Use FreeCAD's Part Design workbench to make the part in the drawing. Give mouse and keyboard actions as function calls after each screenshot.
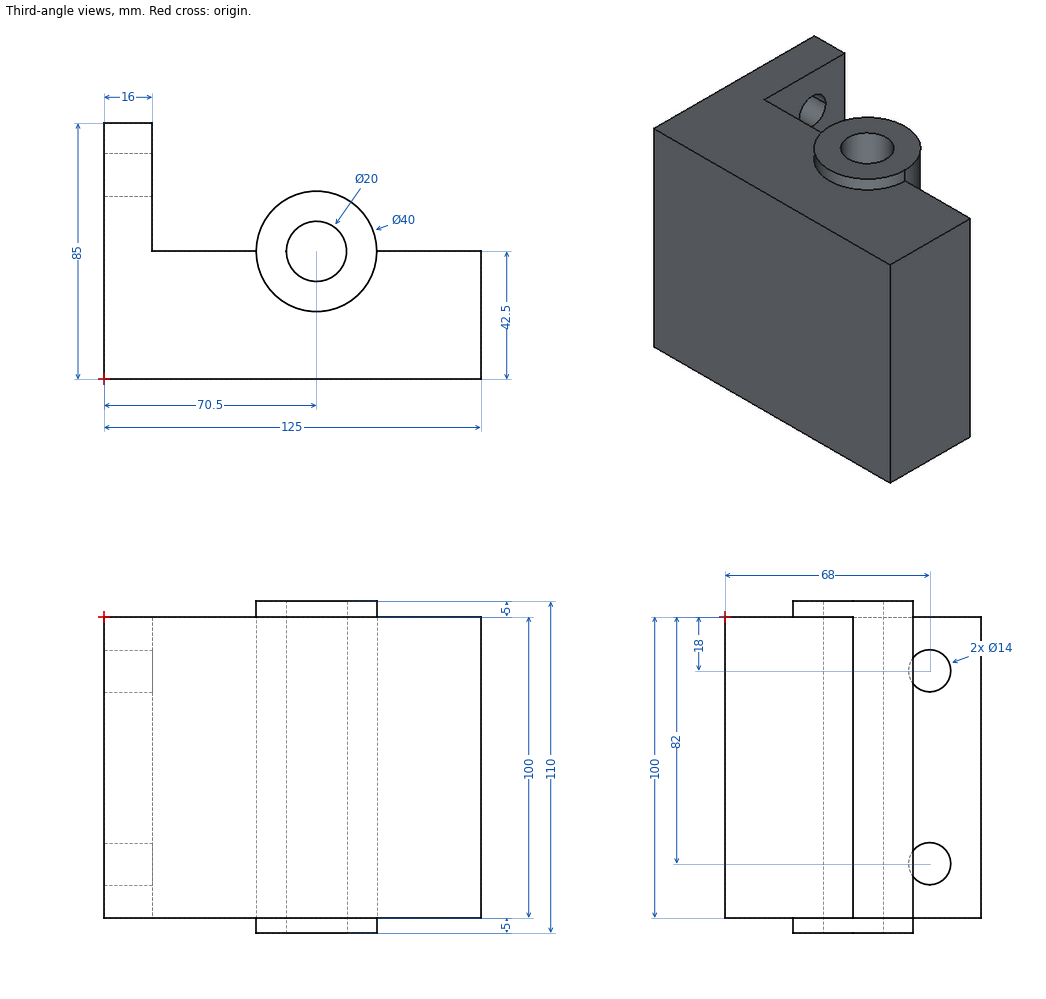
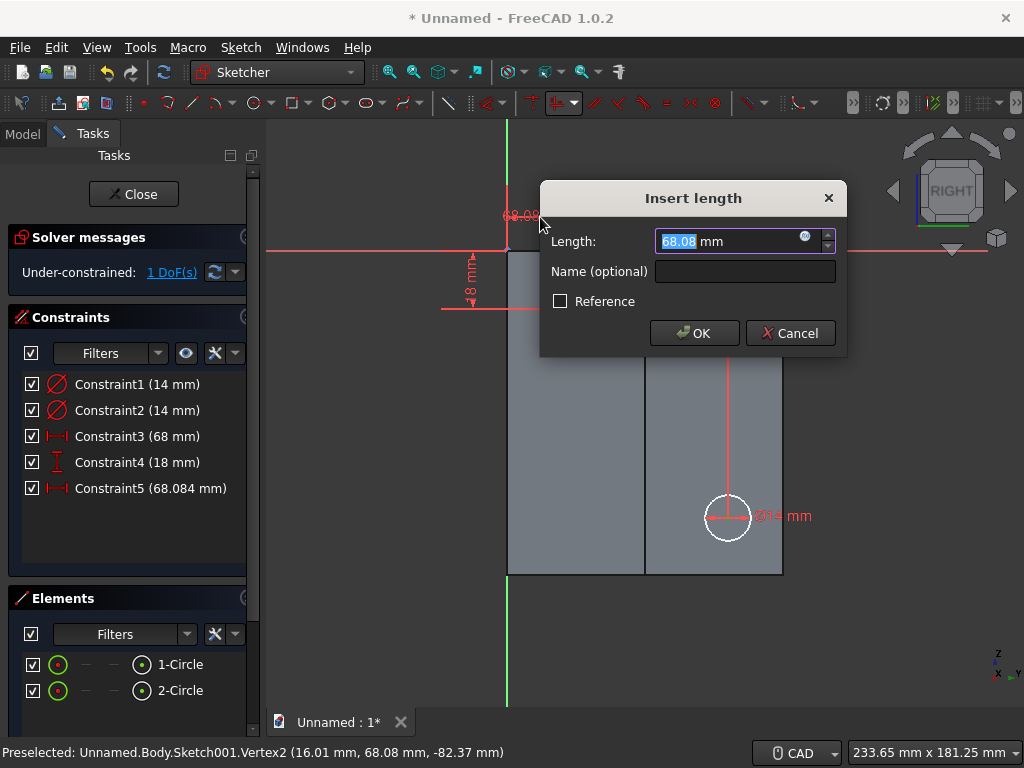
text(68)
key(Return)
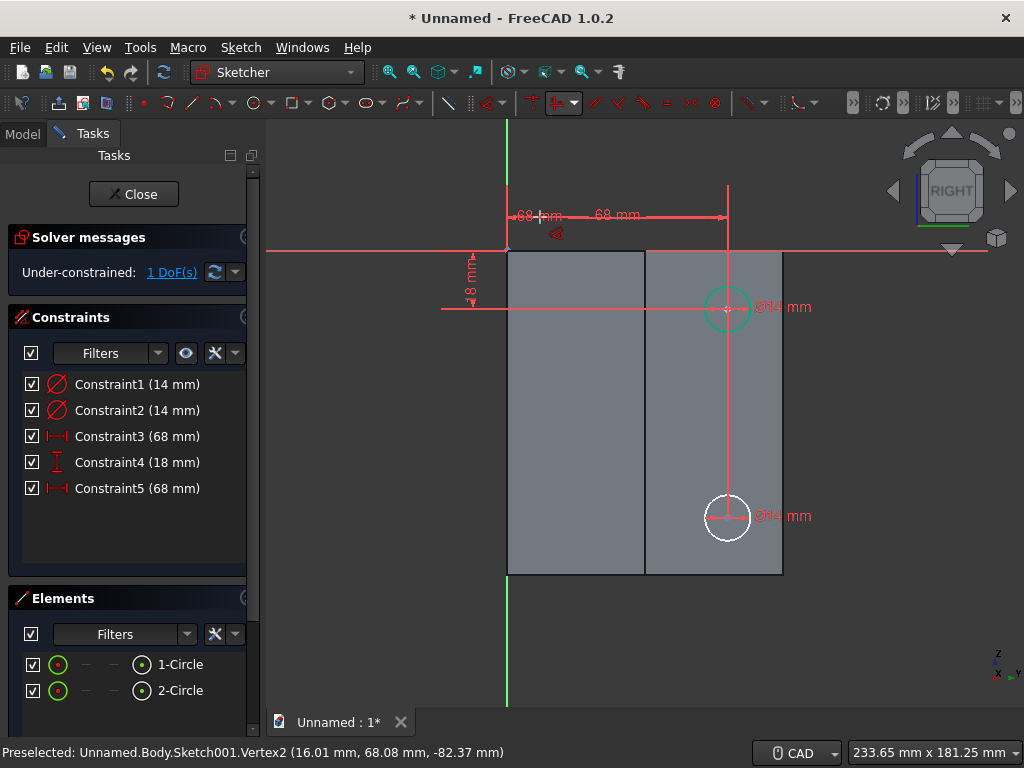
click(728, 518)
click(473, 384)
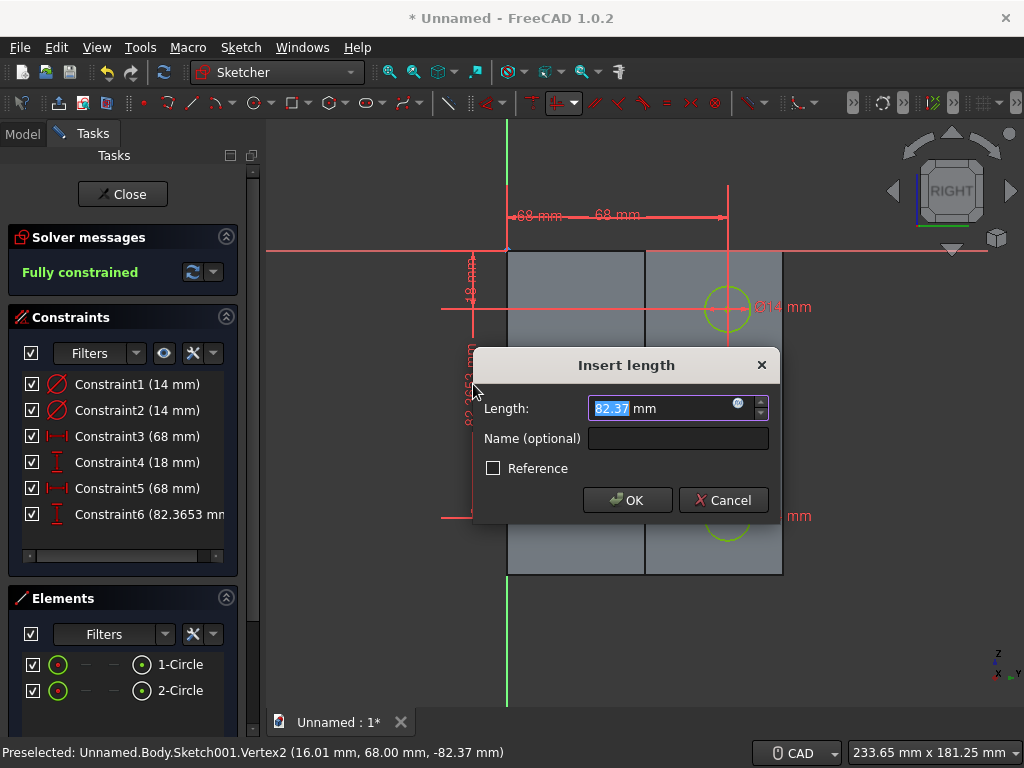
text(82)
key(Return)
key(Escape)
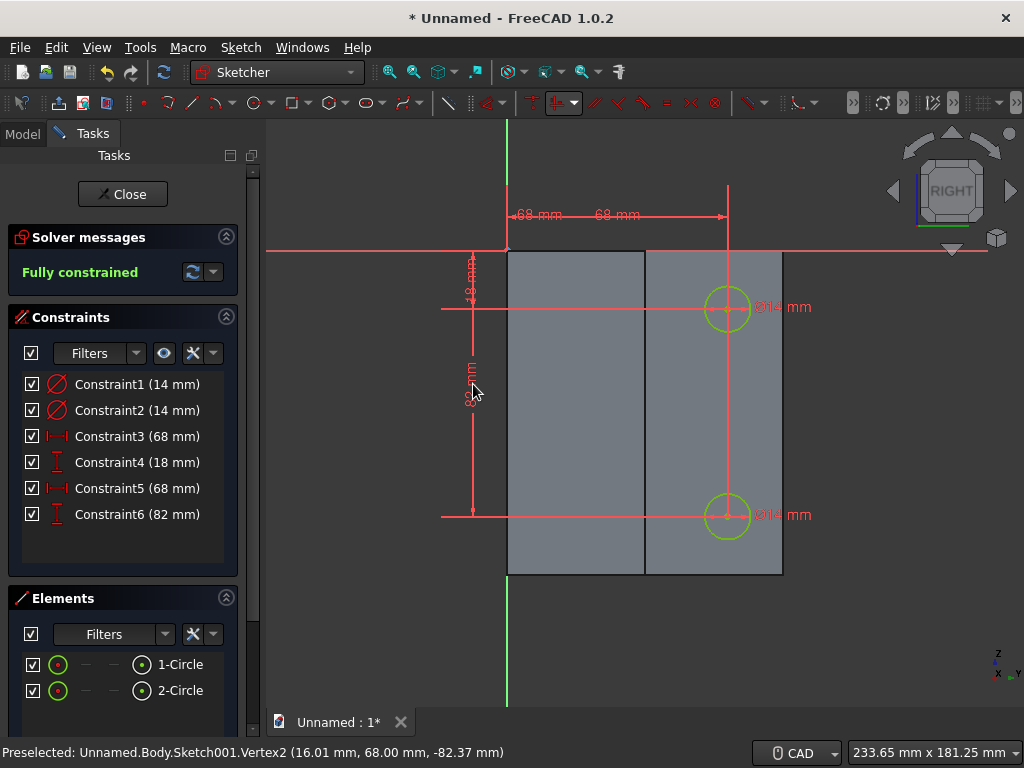
click(123, 194)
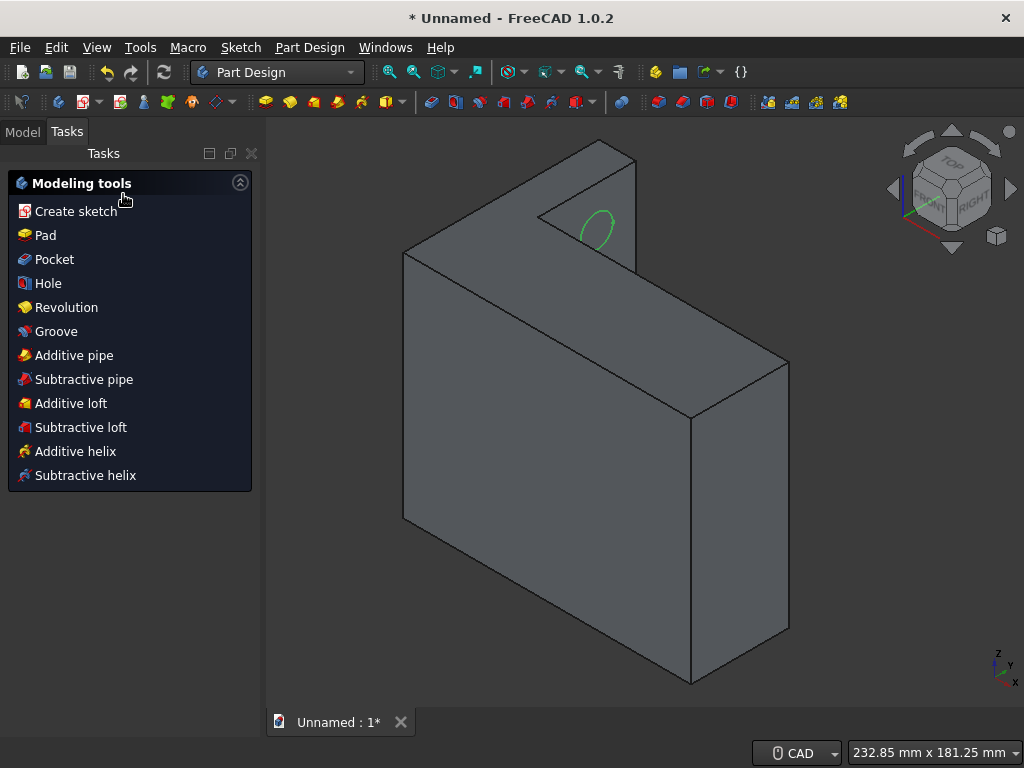
click(432, 102)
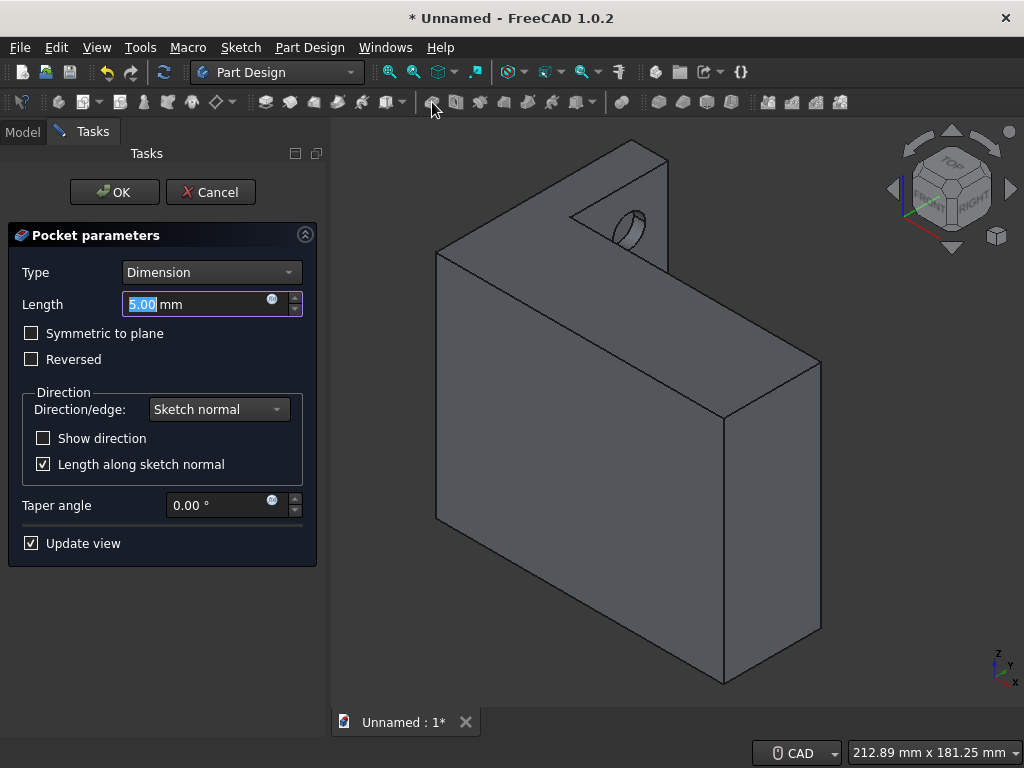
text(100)
key(Tab)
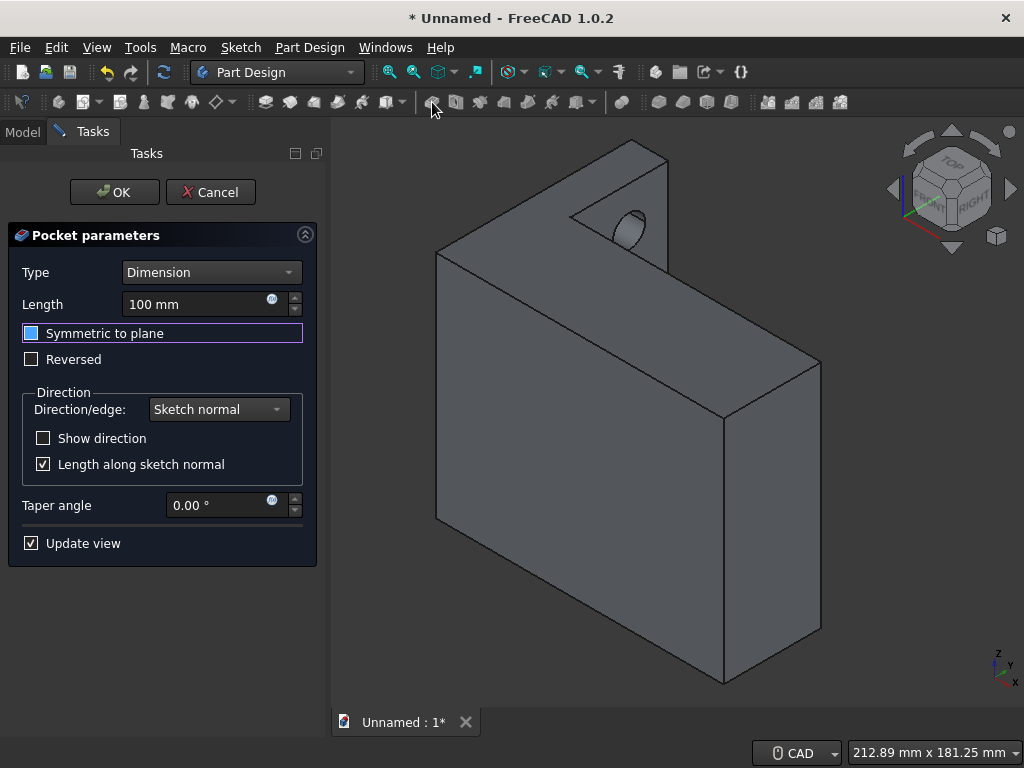
click(115, 192)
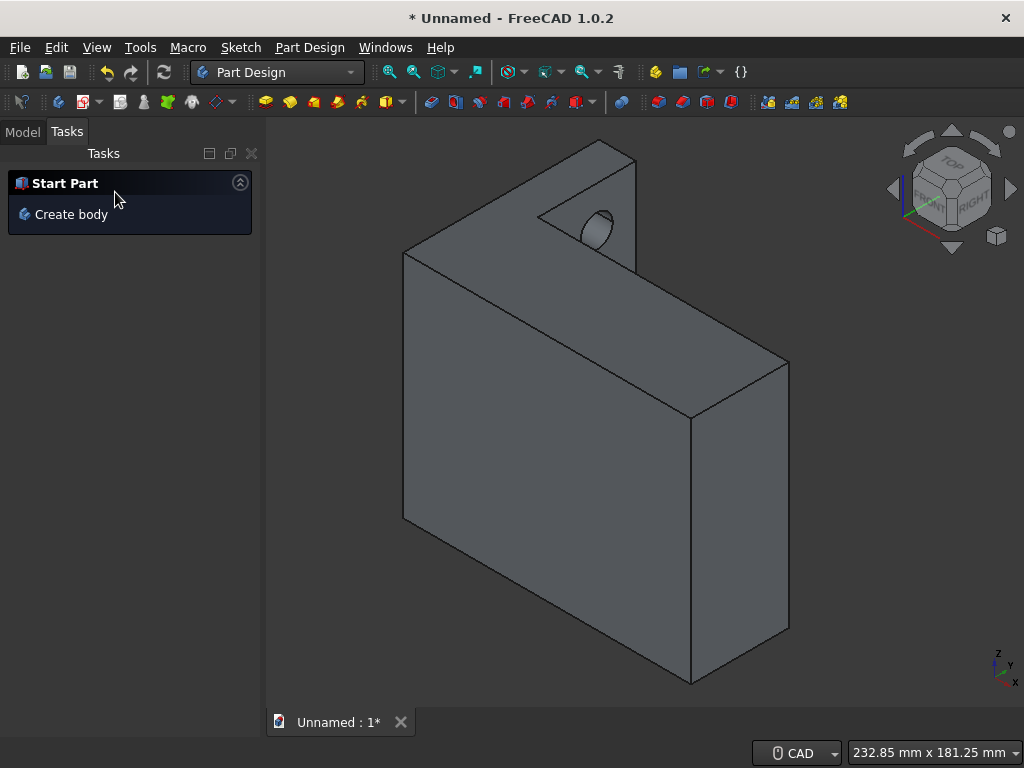
click(84, 102)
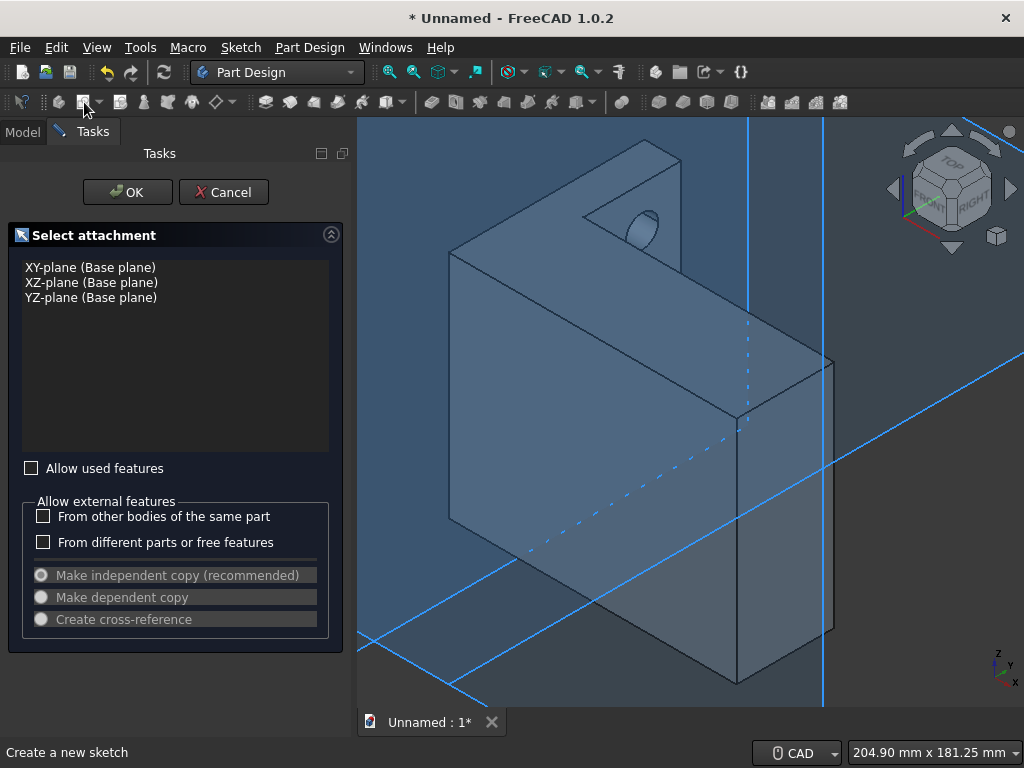
click(82, 268)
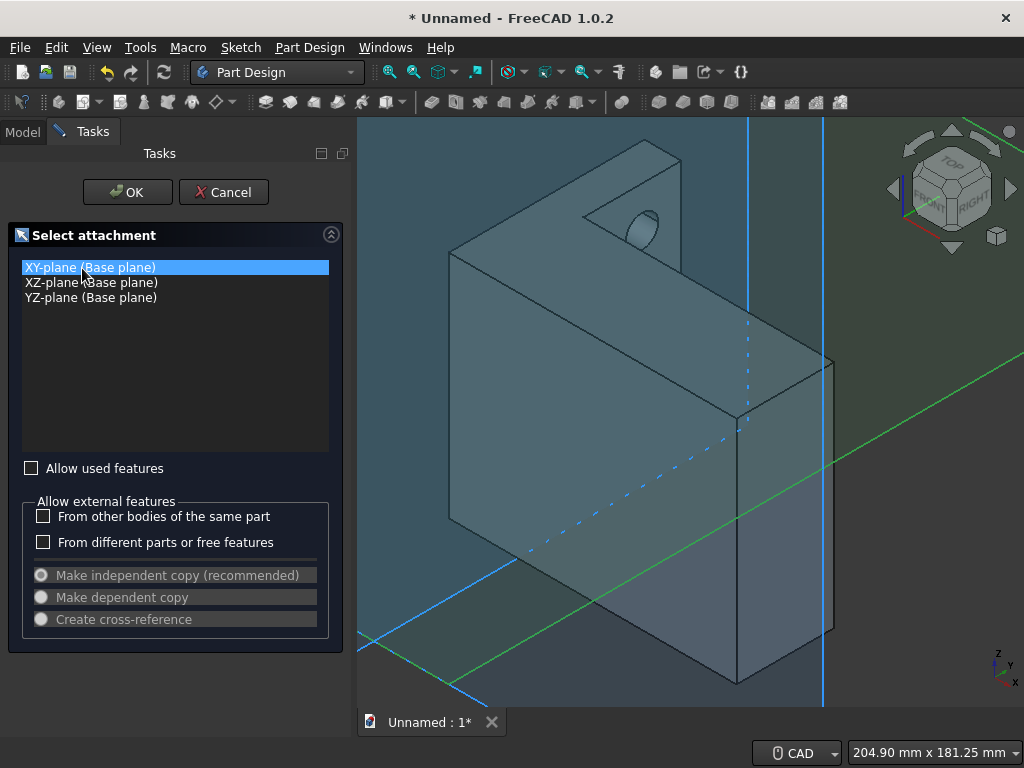
click(128, 192)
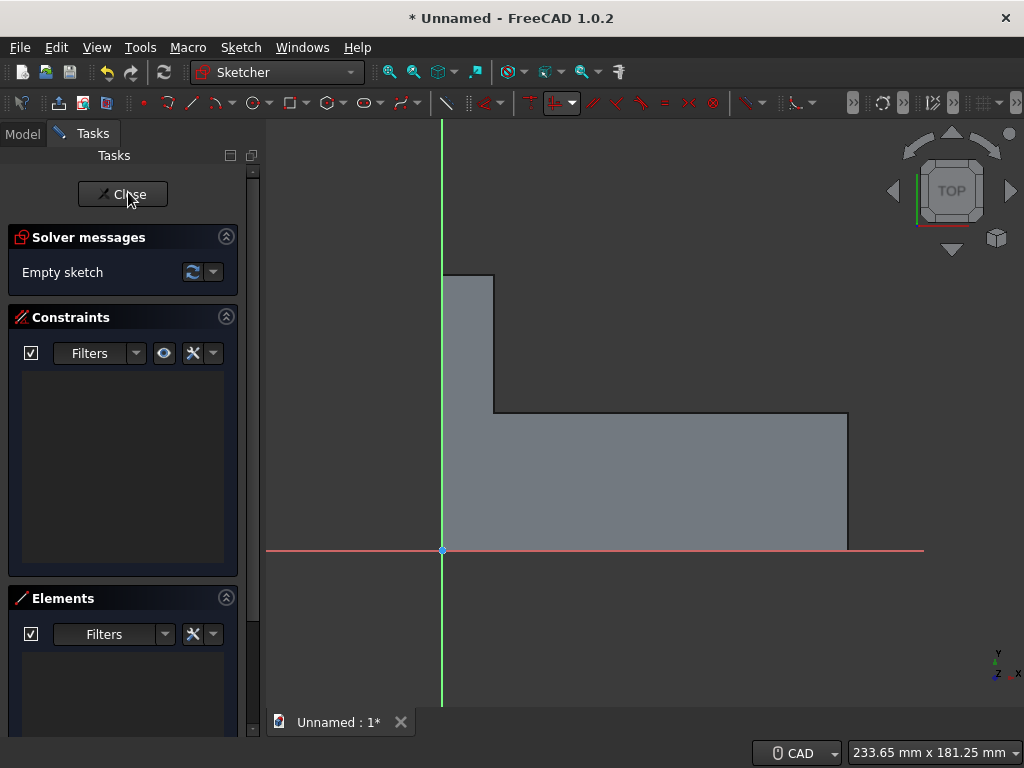
scroll(615, 524, up, 2)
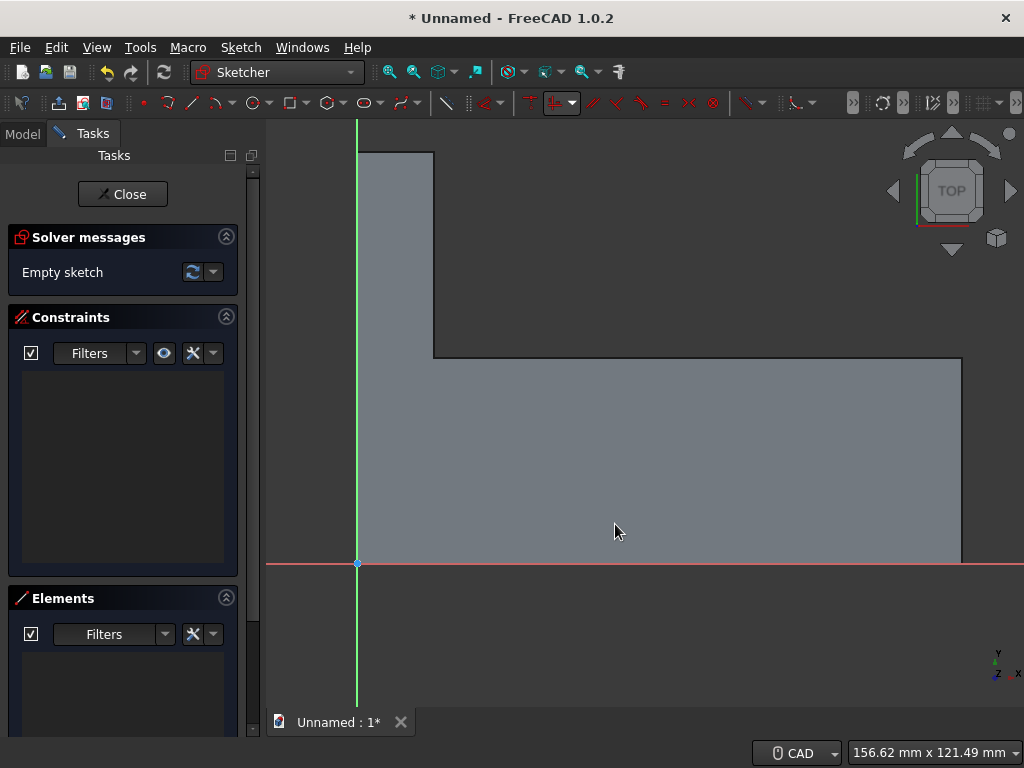
key(g)
key(c)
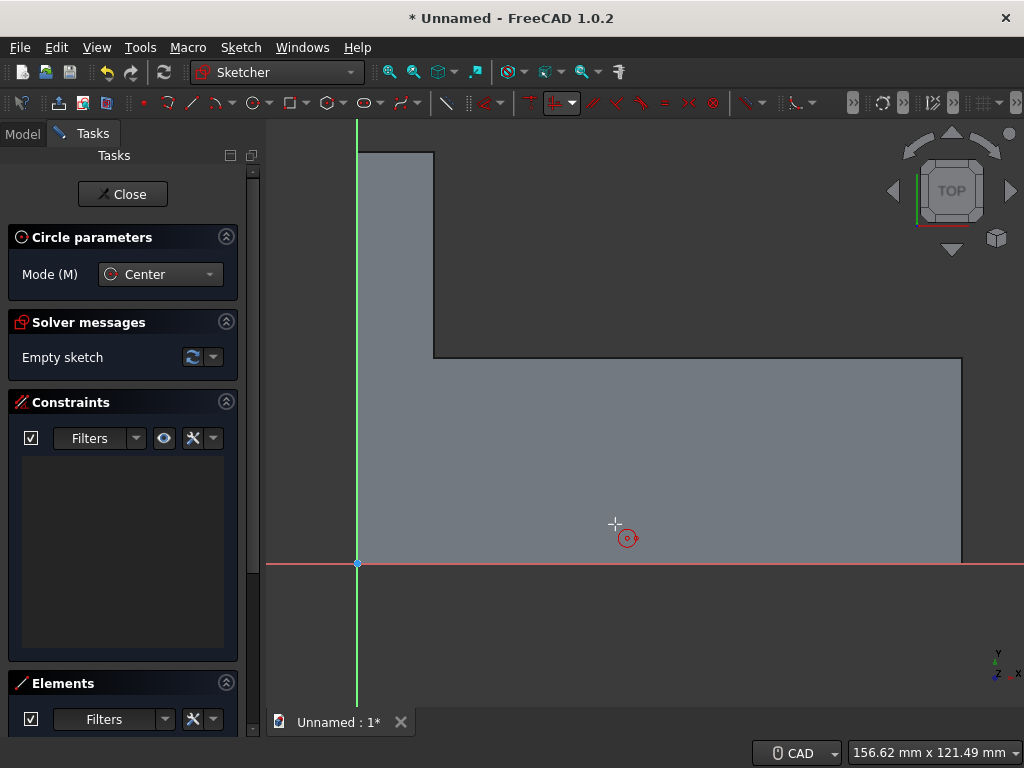
click(698, 358)
move(767, 290)